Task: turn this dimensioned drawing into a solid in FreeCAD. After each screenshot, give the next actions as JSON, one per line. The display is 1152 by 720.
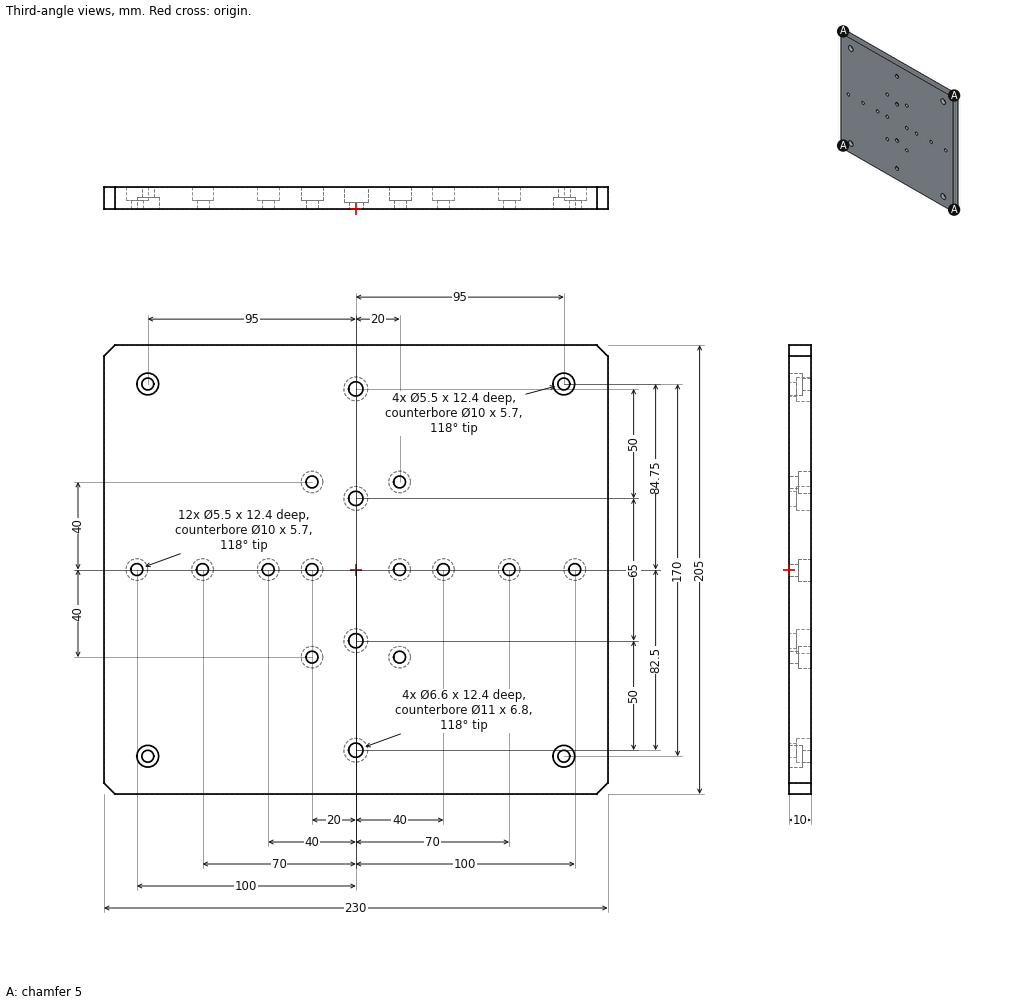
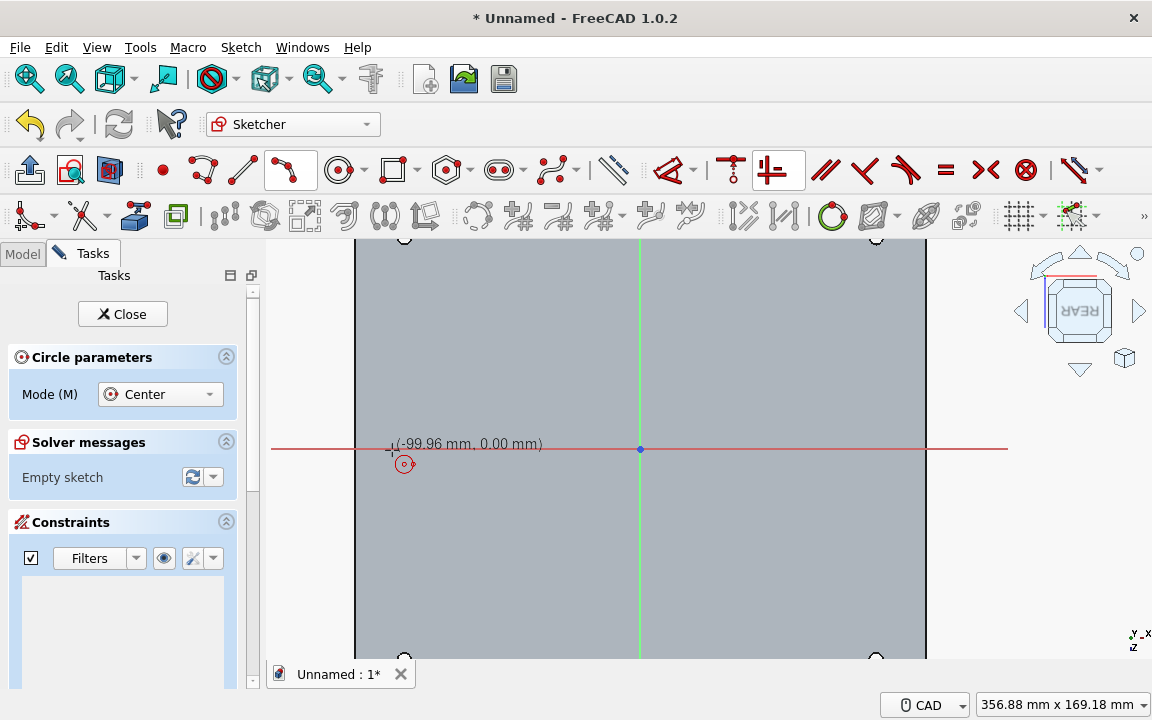
{"action": "left_click", "coordinate": [392, 449]}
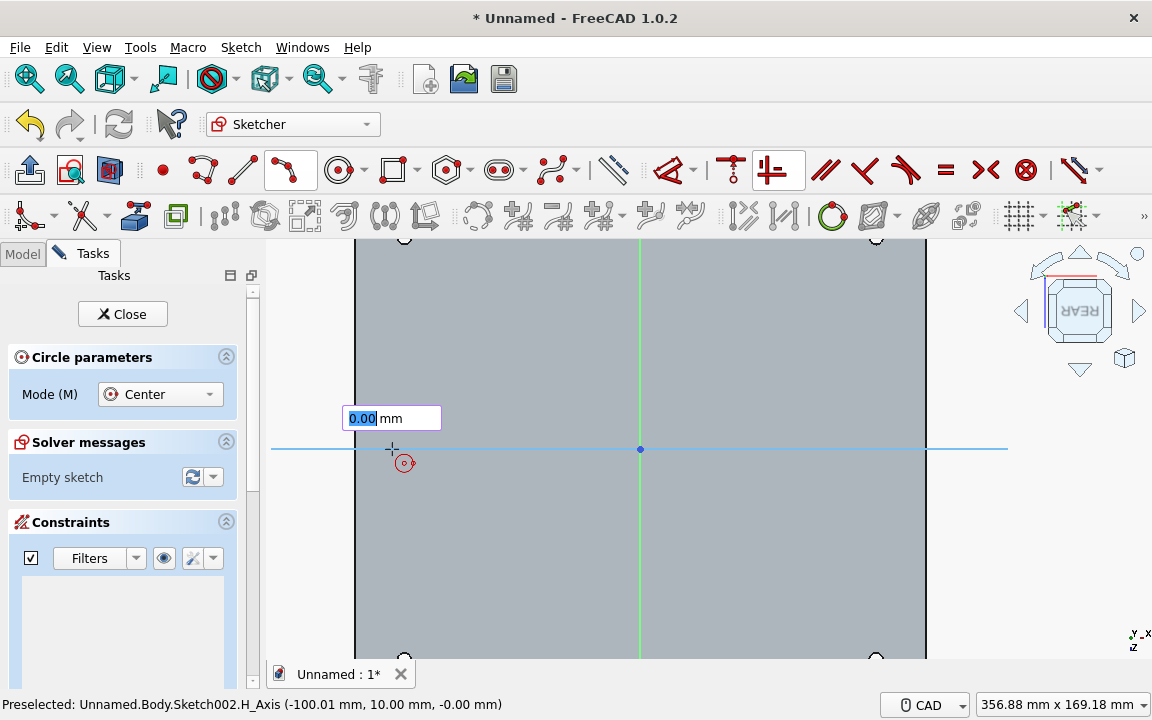
{"action": "scroll", "coordinate": [394, 443], "scroll_direction": "up", "scroll_amount": 5}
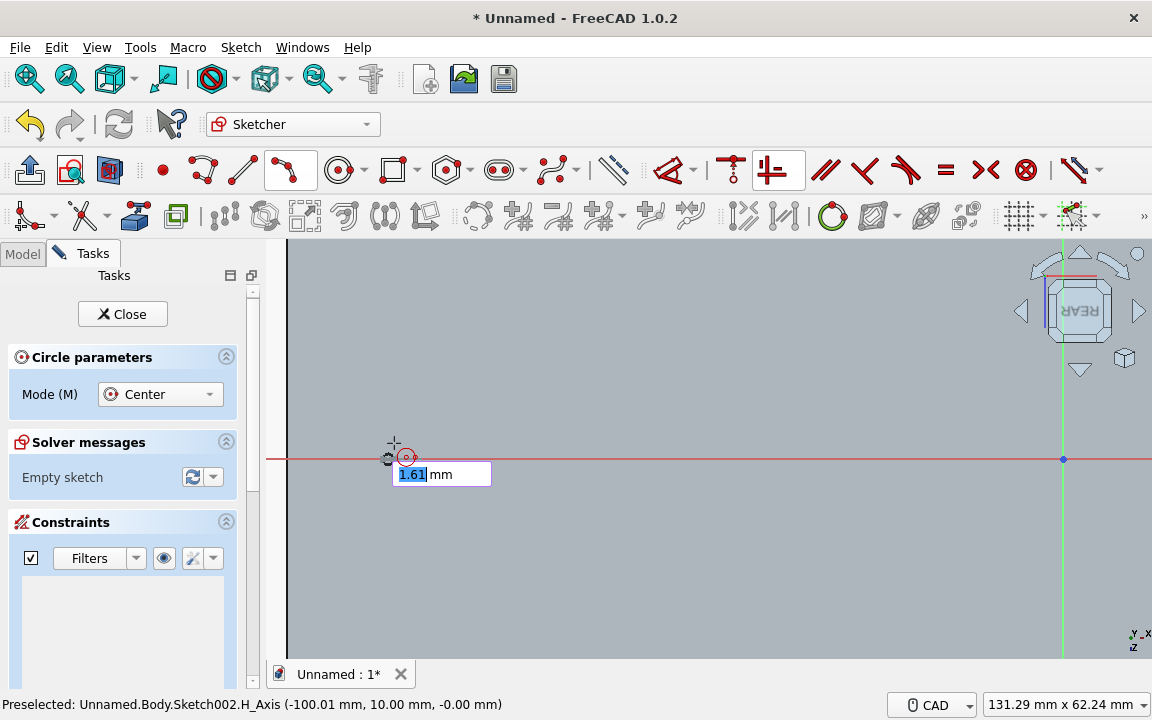
{"action": "left_click", "coordinate": [395, 442]}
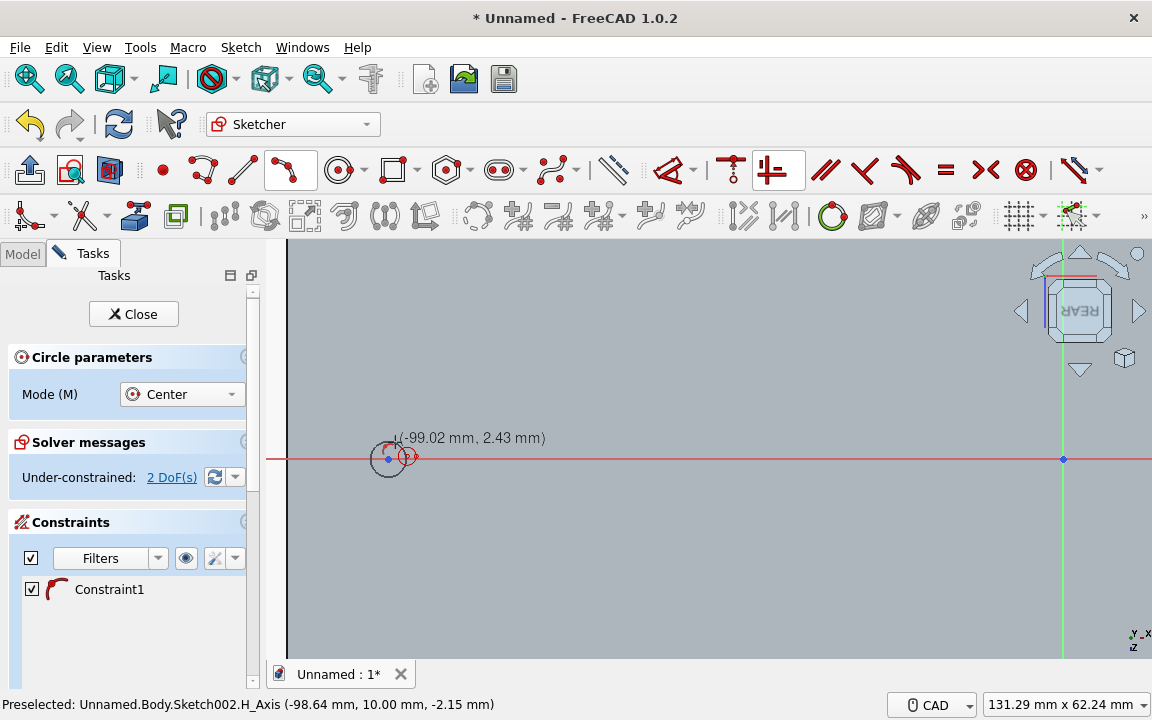
{"action": "scroll", "coordinate": [591, 459], "scroll_direction": "up", "scroll_amount": 2}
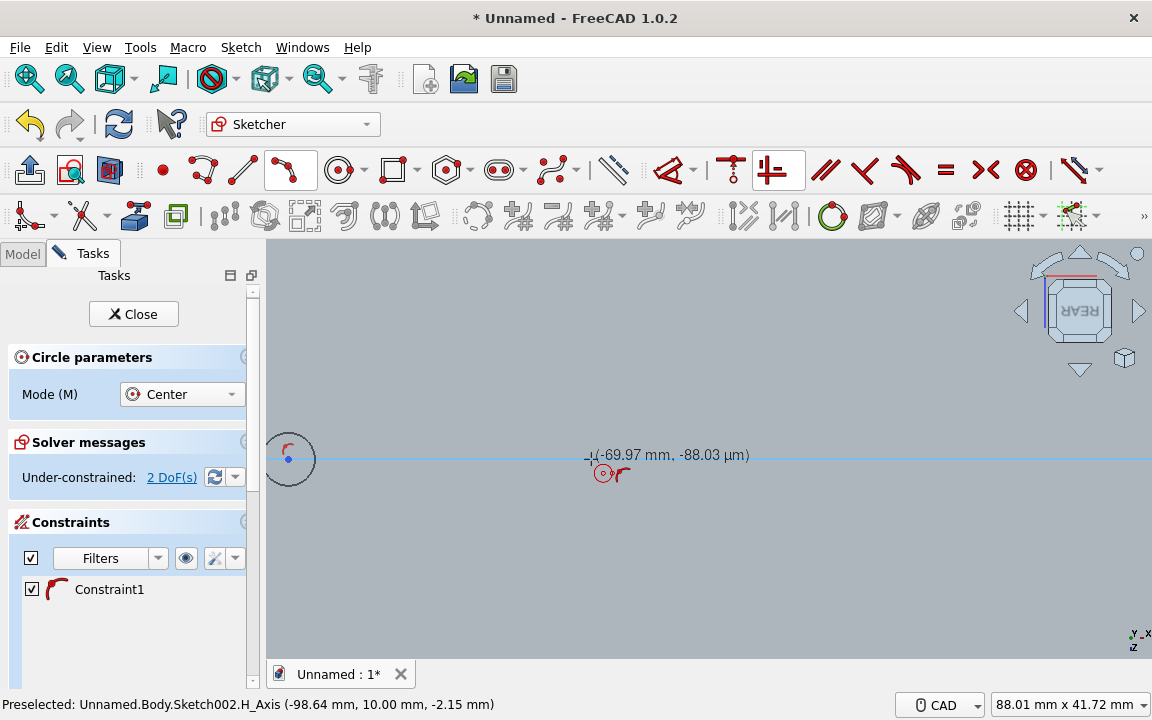
{"action": "scroll", "coordinate": [426, 446], "scroll_direction": "down", "scroll_amount": 7}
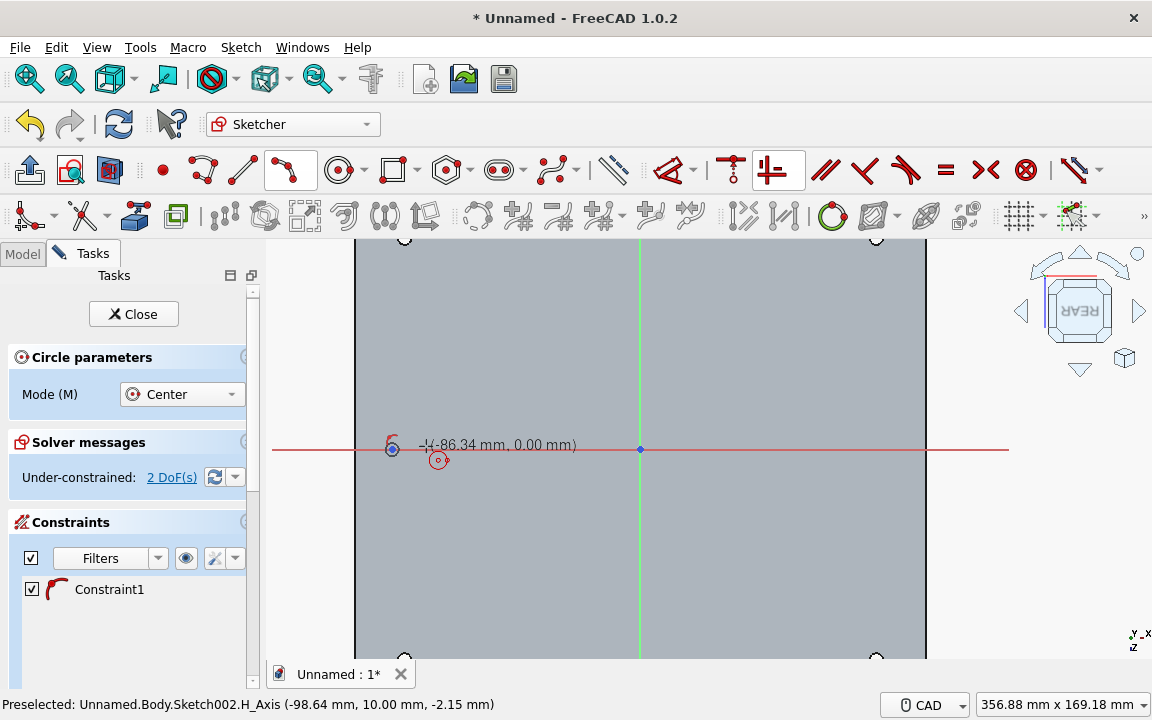
{"action": "left_click", "coordinate": [467, 450]}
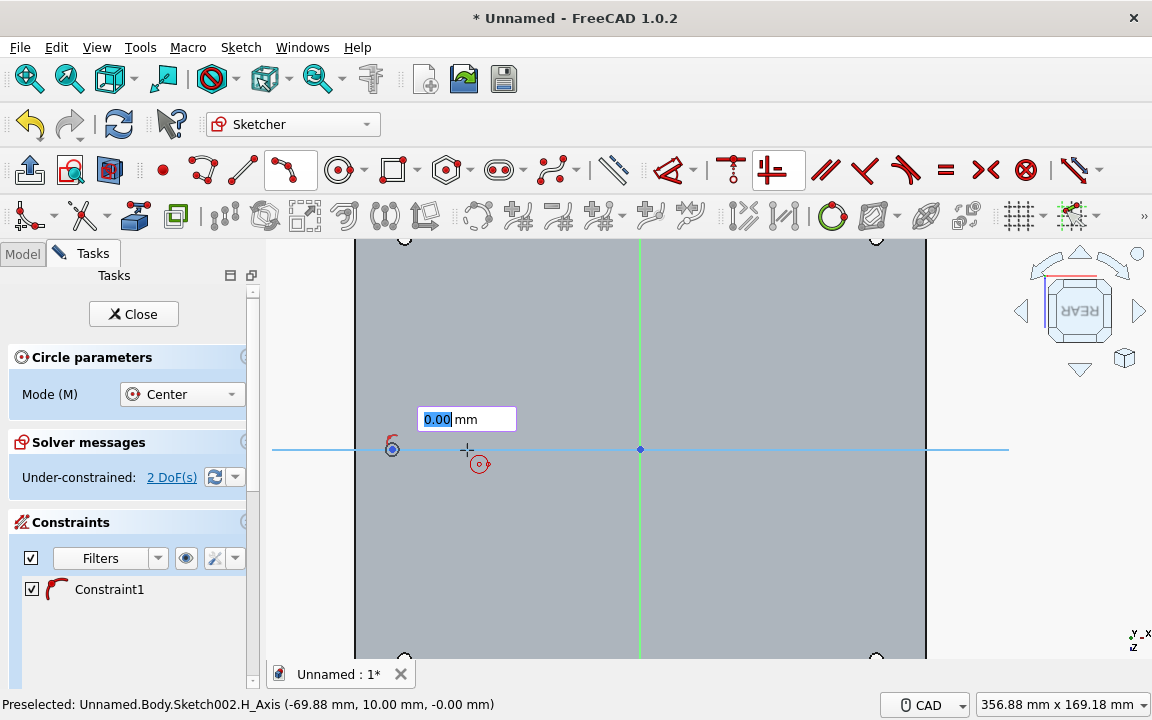
{"action": "scroll", "coordinate": [469, 443], "scroll_direction": "up", "scroll_amount": 5}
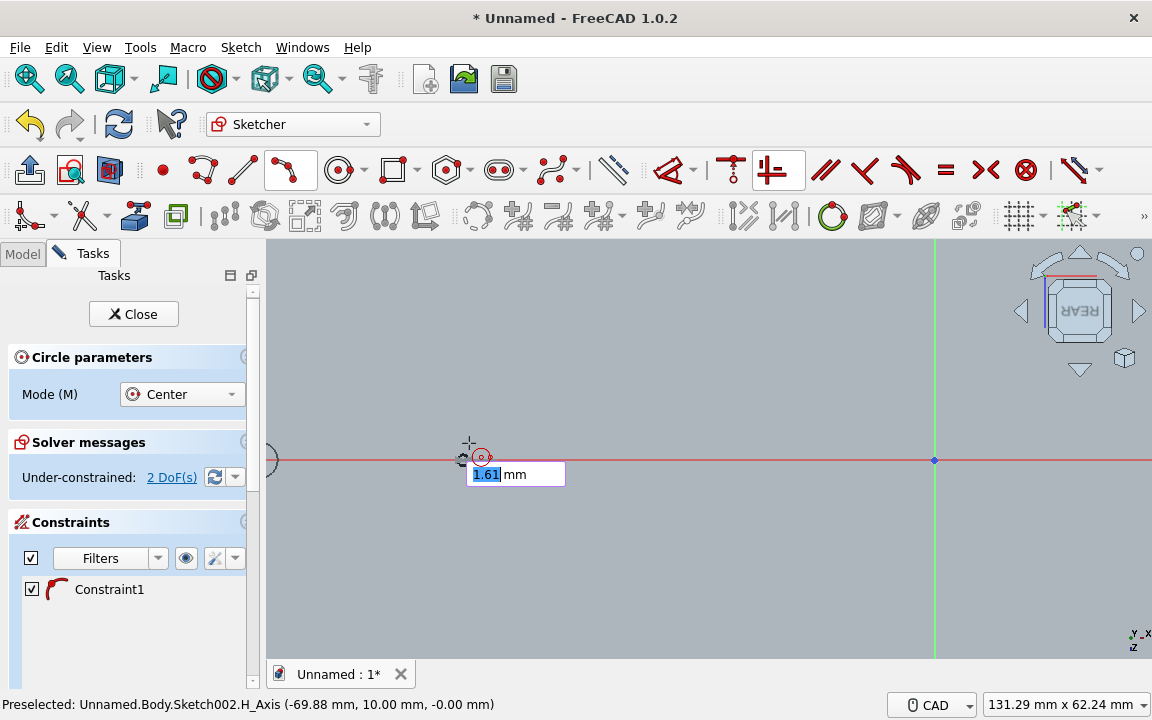
{"action": "left_click", "coordinate": [469, 443]}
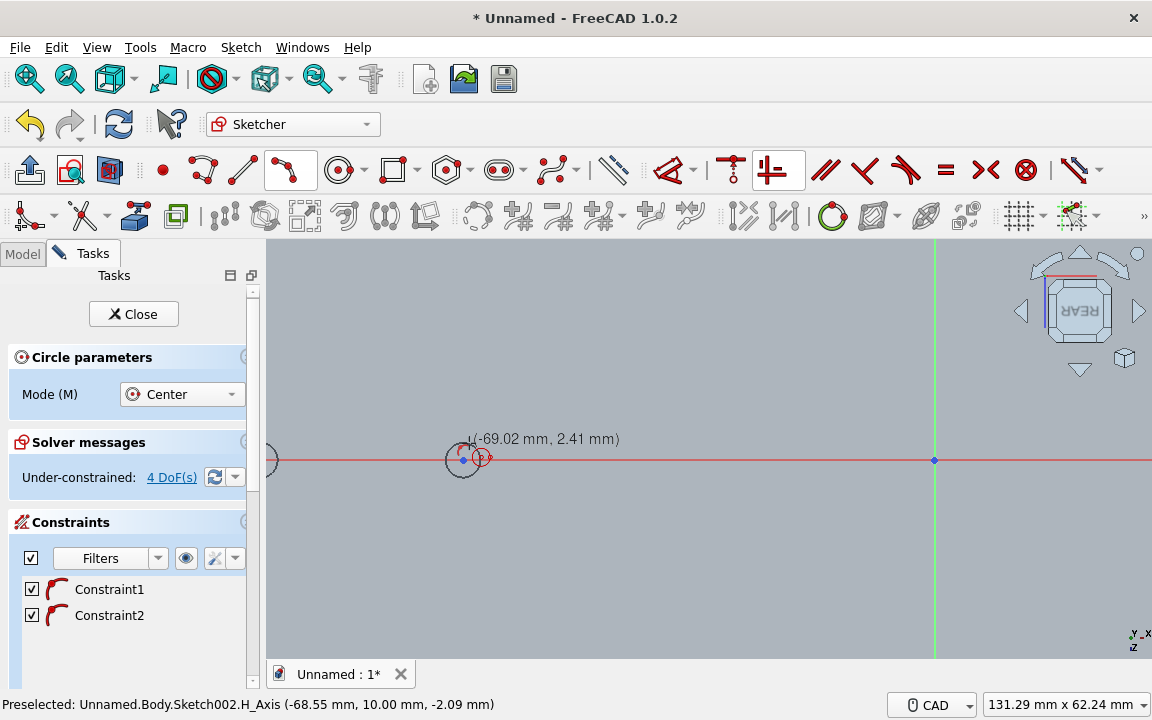
{"action": "scroll", "coordinate": [665, 460], "scroll_direction": "up", "scroll_amount": 2}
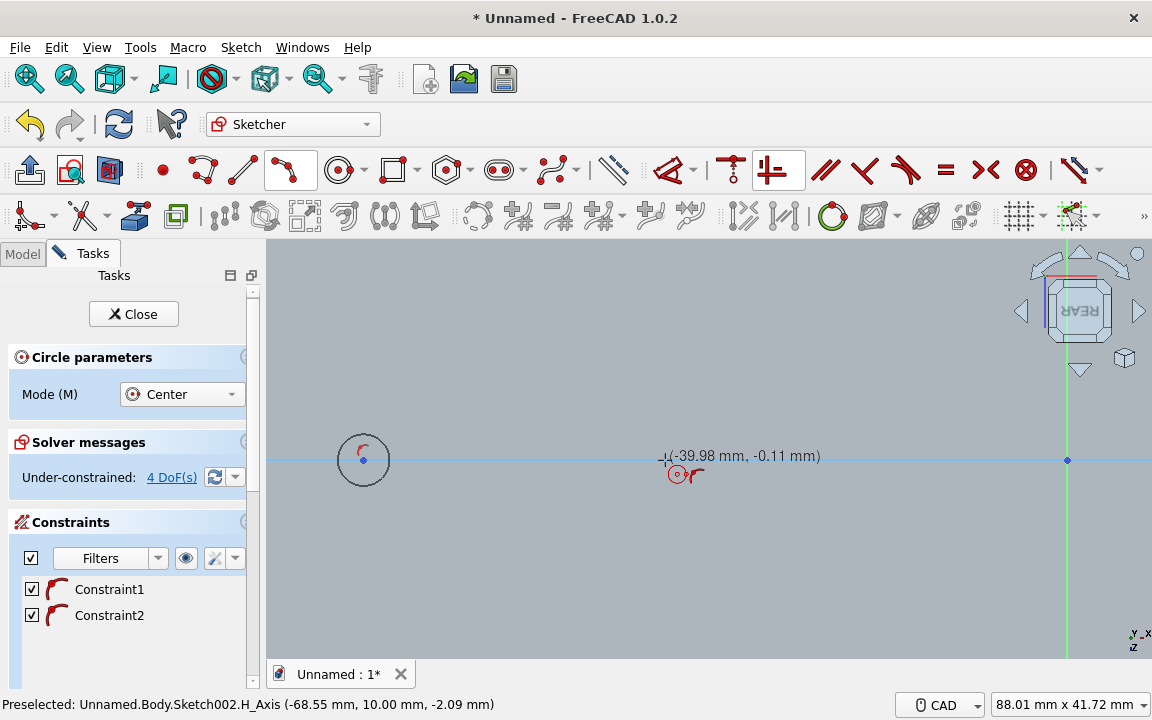
{"action": "scroll", "coordinate": [501, 445], "scroll_direction": "down", "scroll_amount": 7}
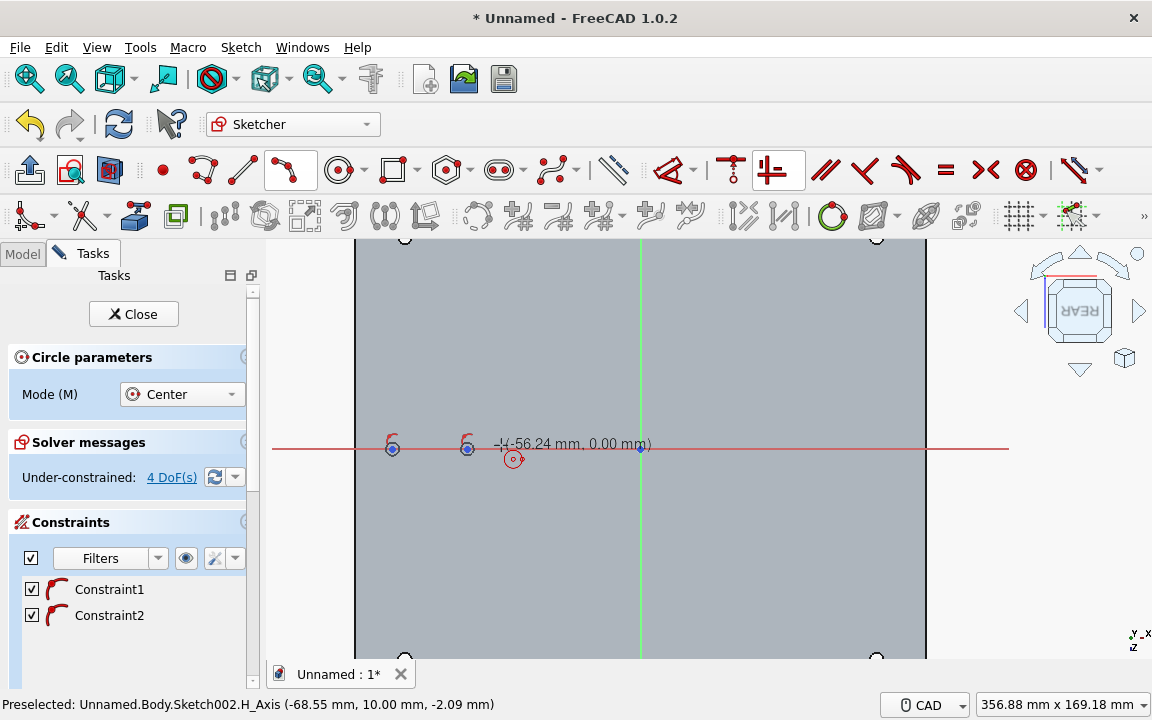
{"action": "left_click", "coordinate": [542, 449]}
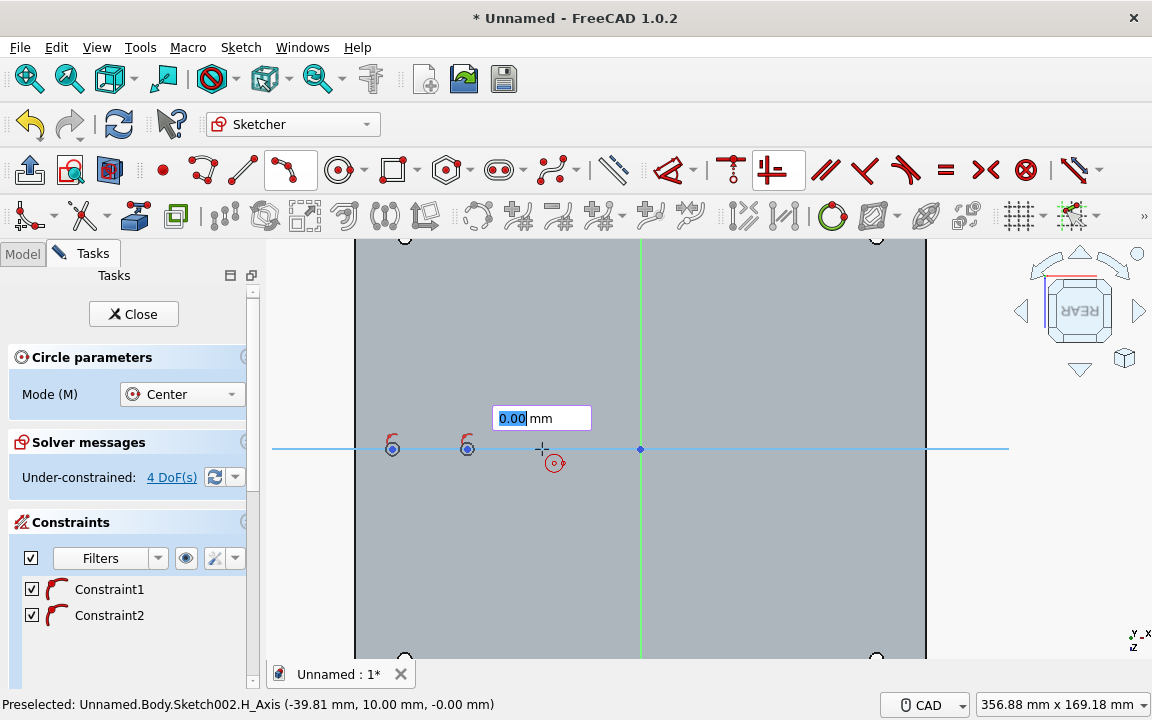
{"action": "scroll", "coordinate": [544, 443], "scroll_direction": "up", "scroll_amount": 5}